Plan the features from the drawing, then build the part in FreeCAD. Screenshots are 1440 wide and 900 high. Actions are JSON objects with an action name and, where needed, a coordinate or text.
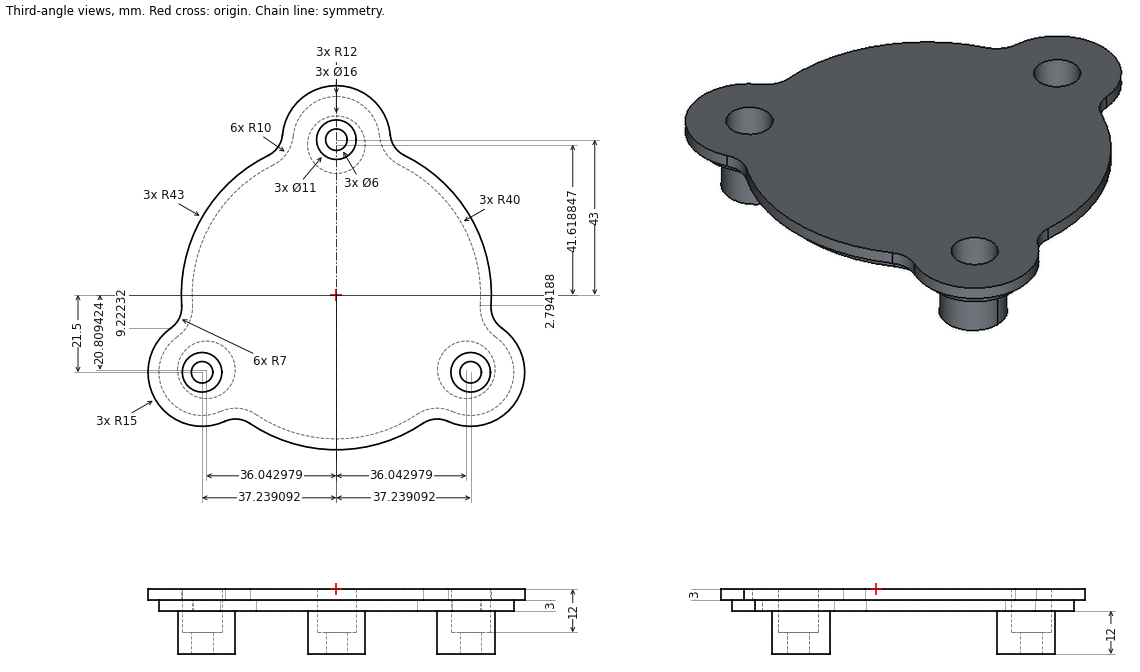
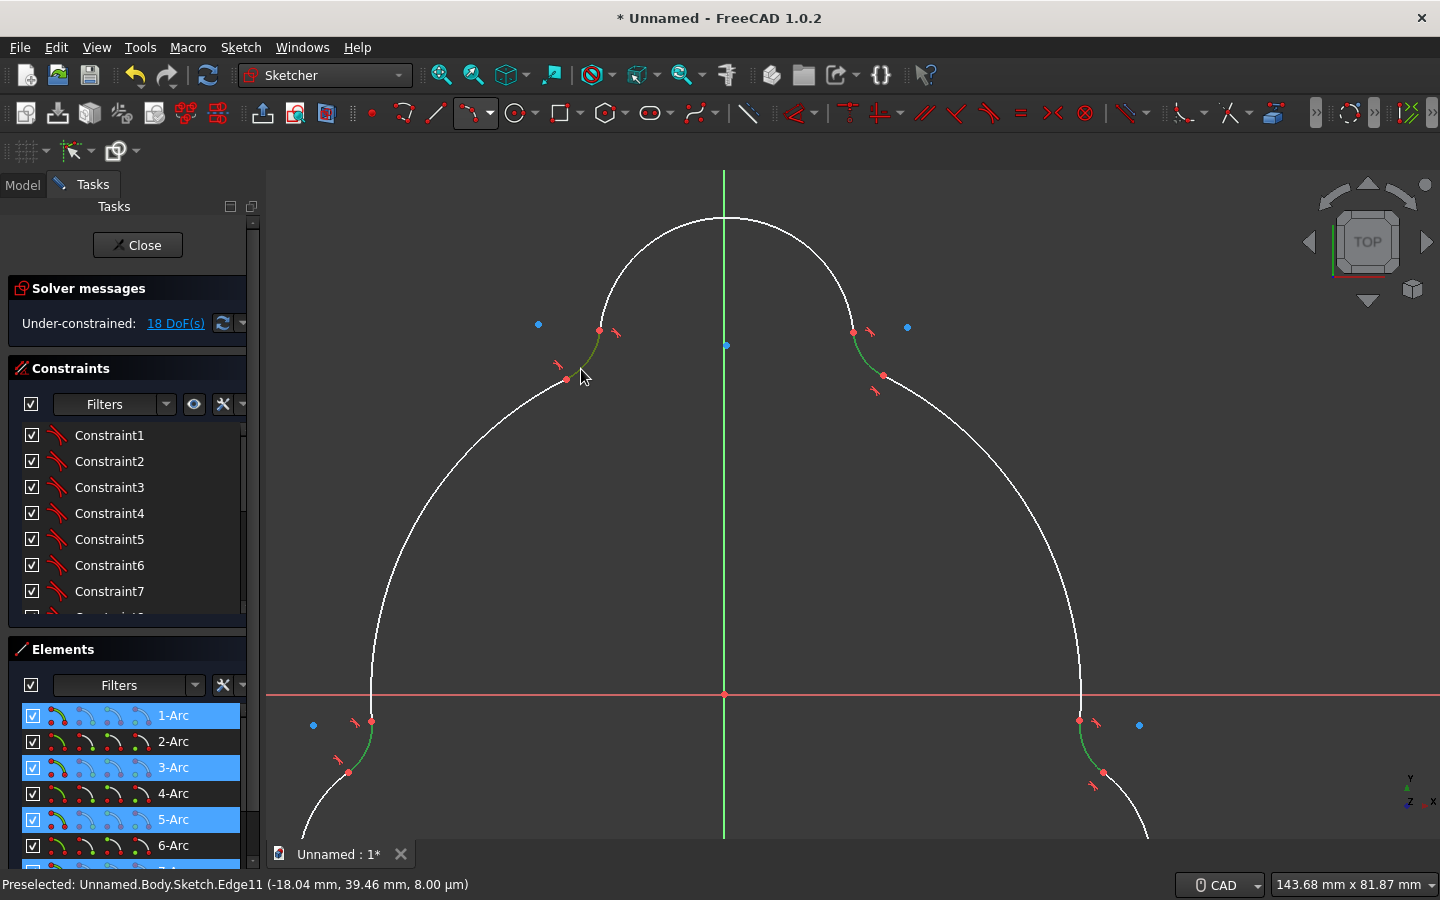
{"action": "left_click", "coordinate": [1022, 114]}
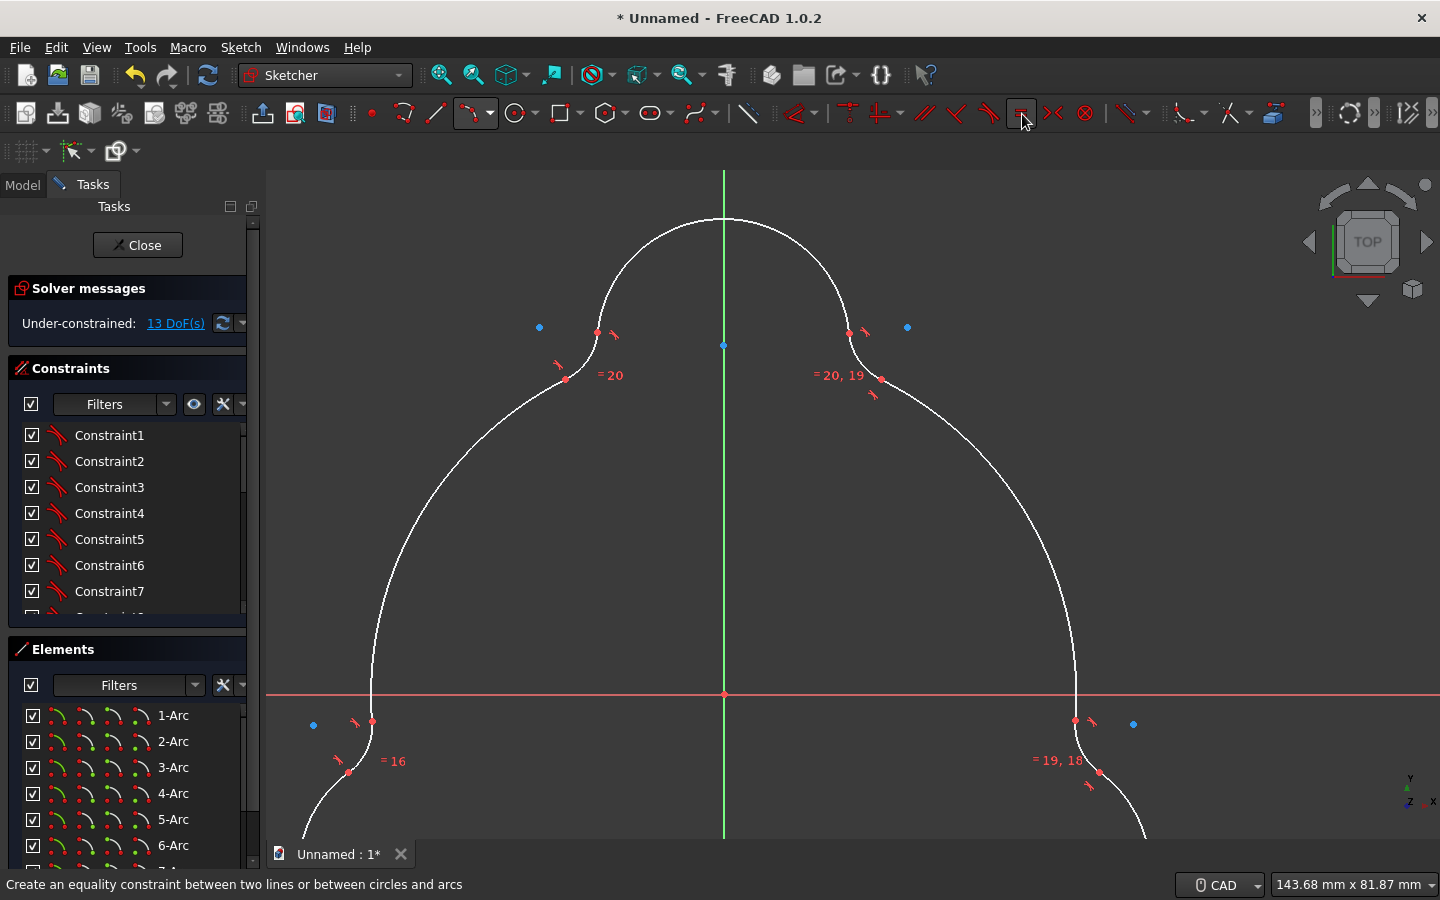
{"action": "scroll", "coordinate": [858, 347], "scroll_direction": "down", "scroll_amount": 3}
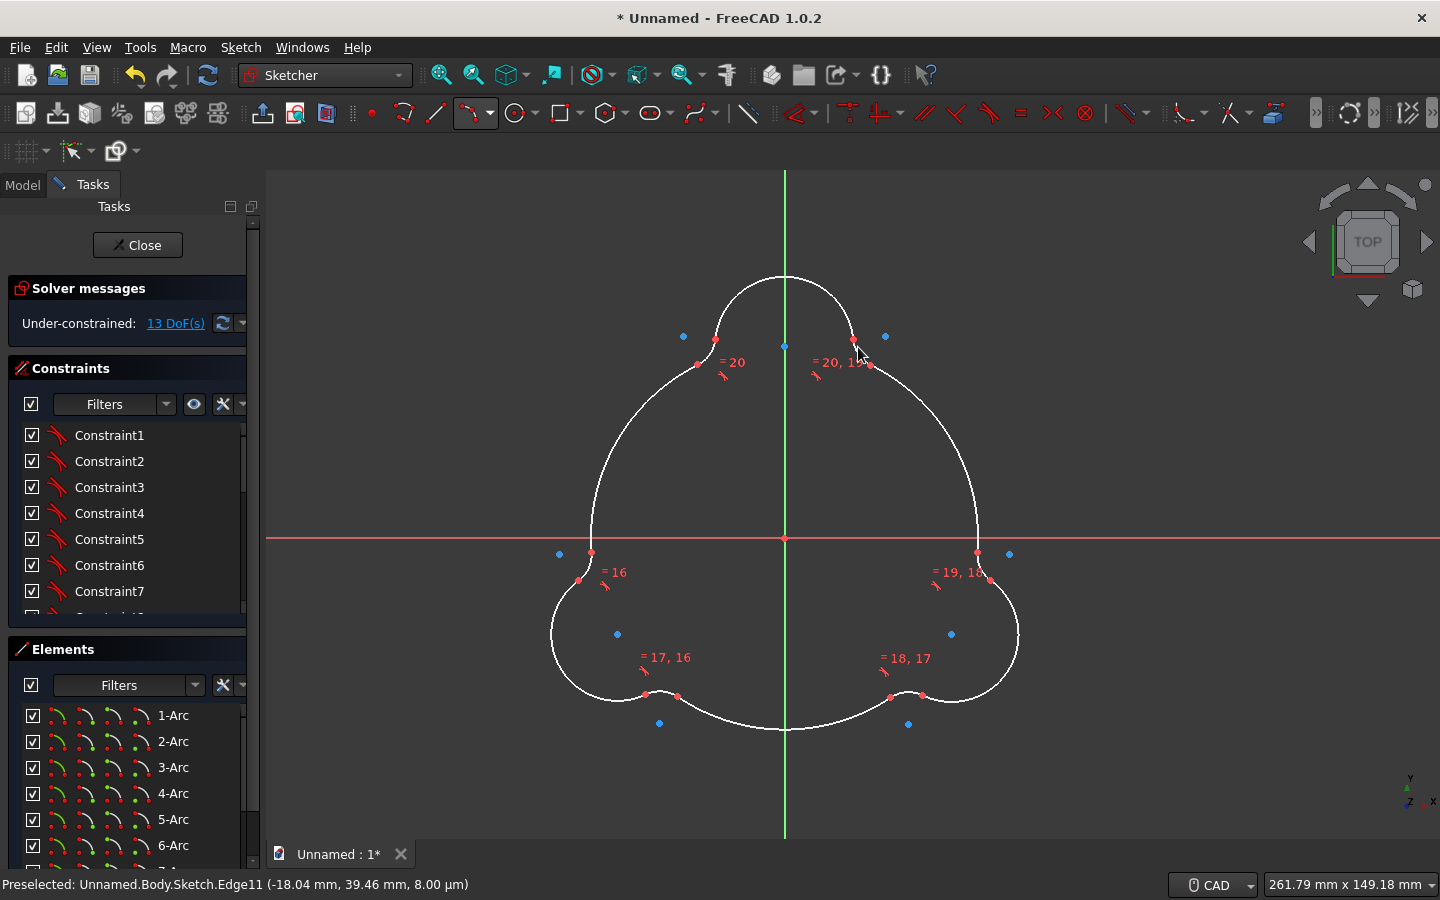
{"action": "left_click", "coordinate": [551, 631]}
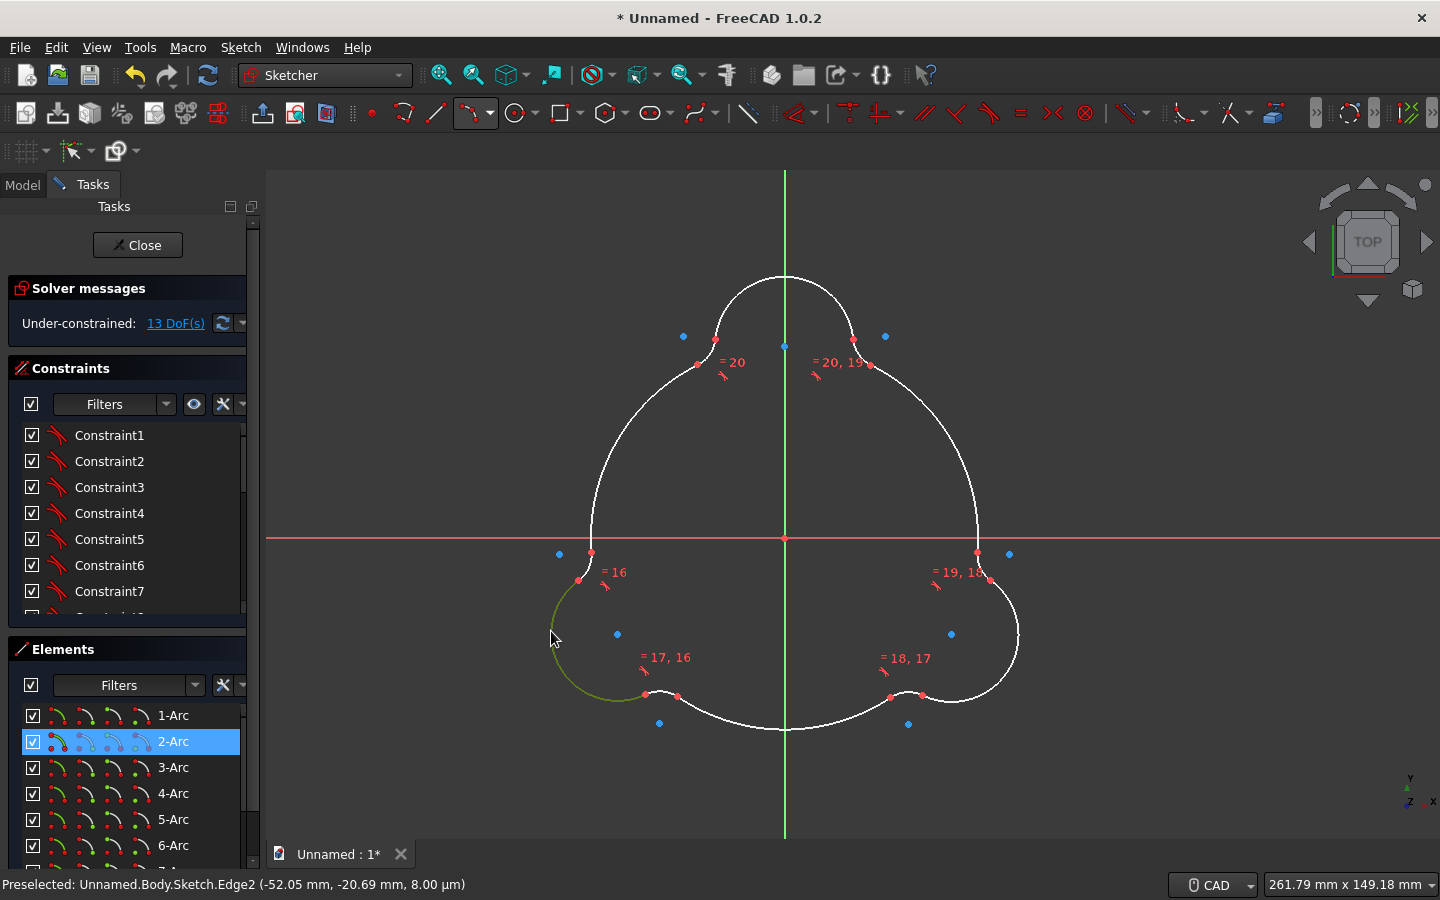
{"action": "left_click", "coordinate": [980, 695]}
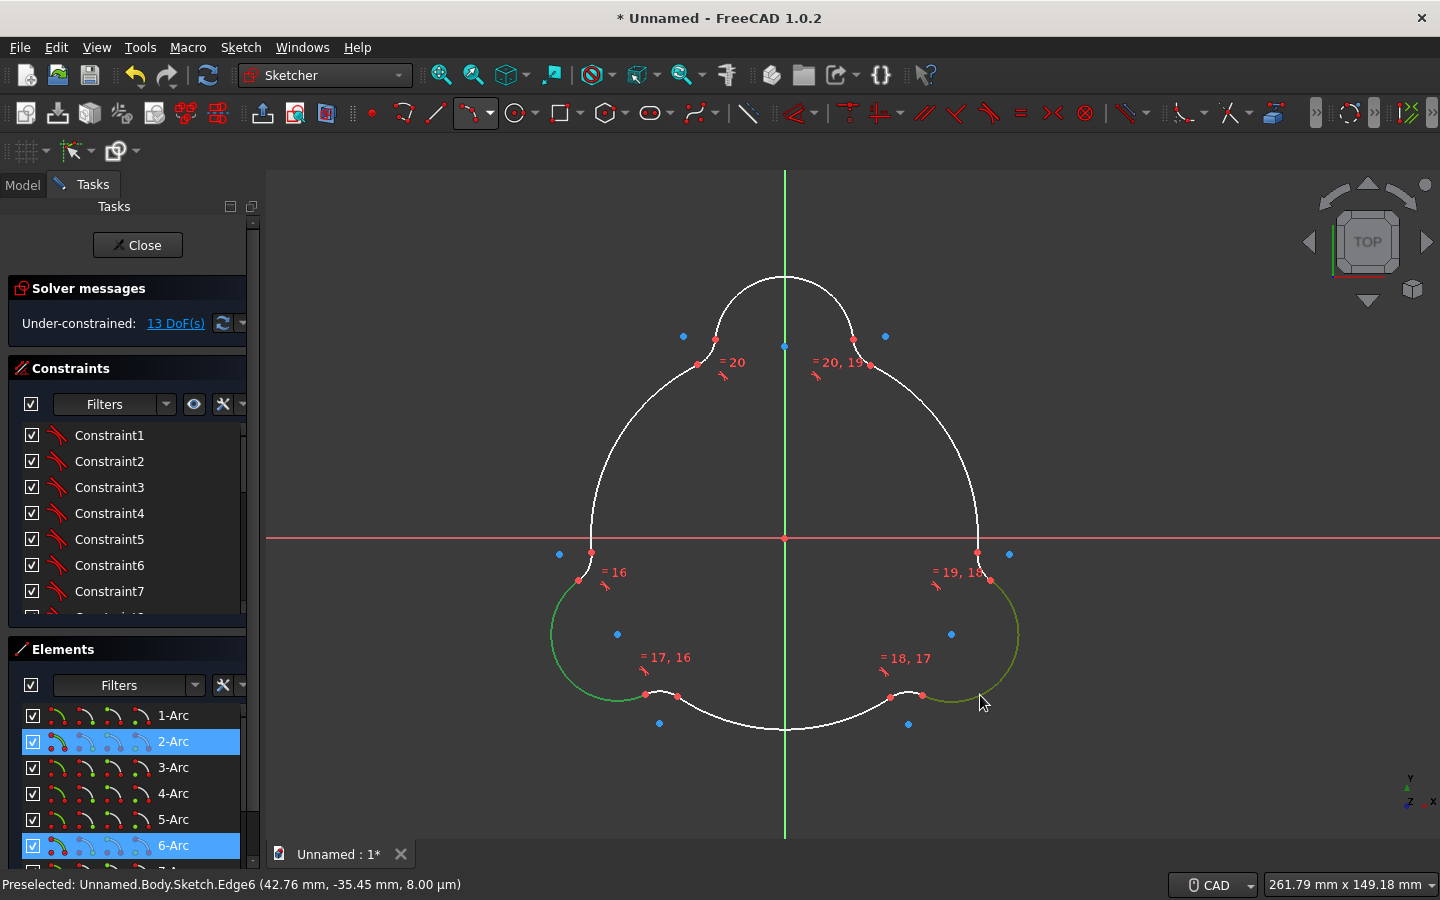
{"action": "left_click", "coordinate": [823, 289]}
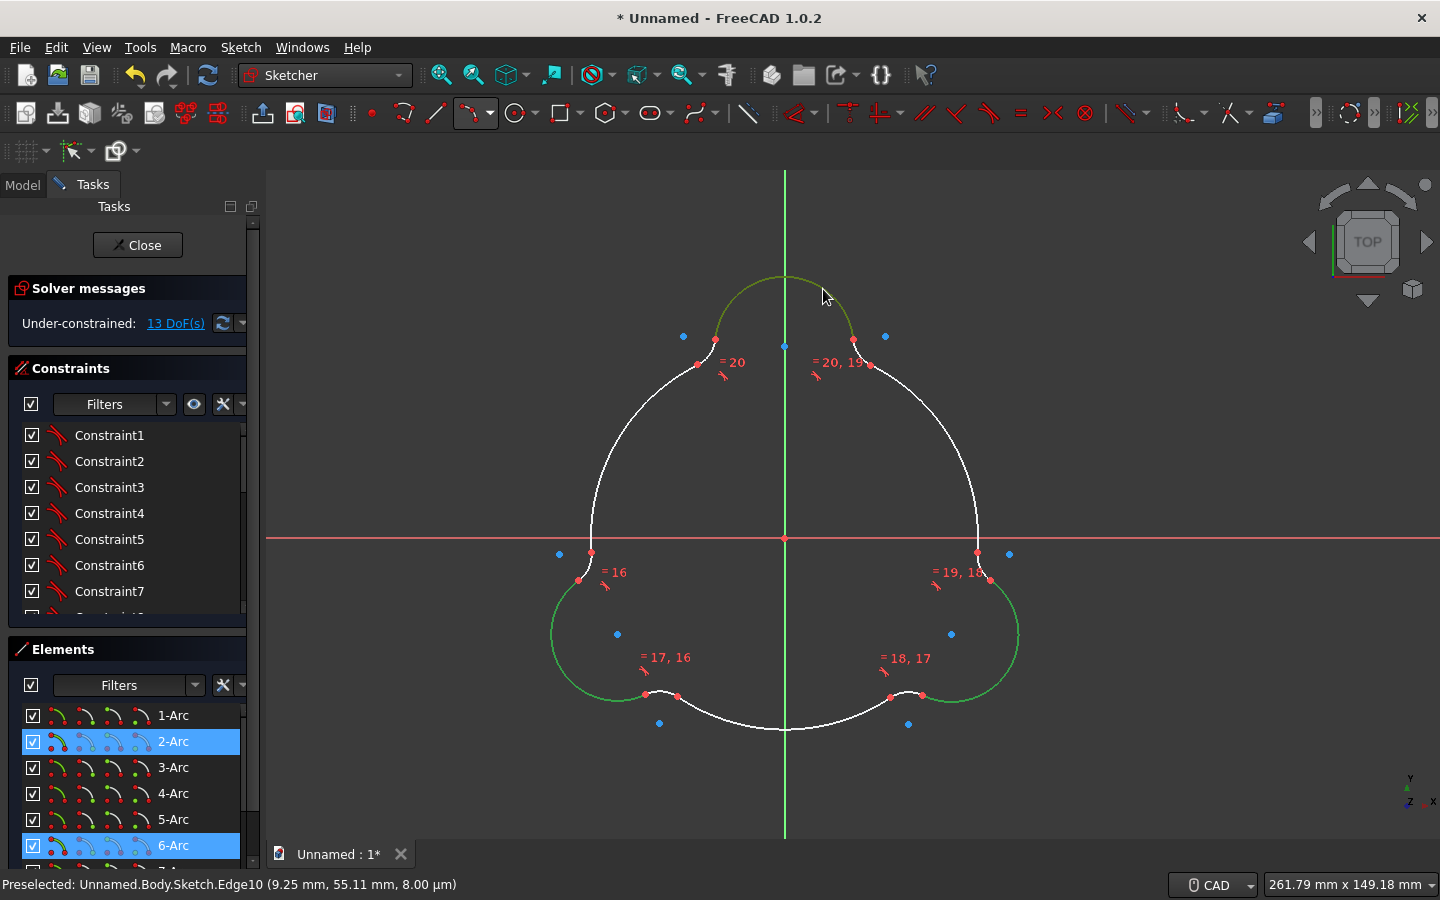
{"action": "left_click", "coordinate": [1022, 114]}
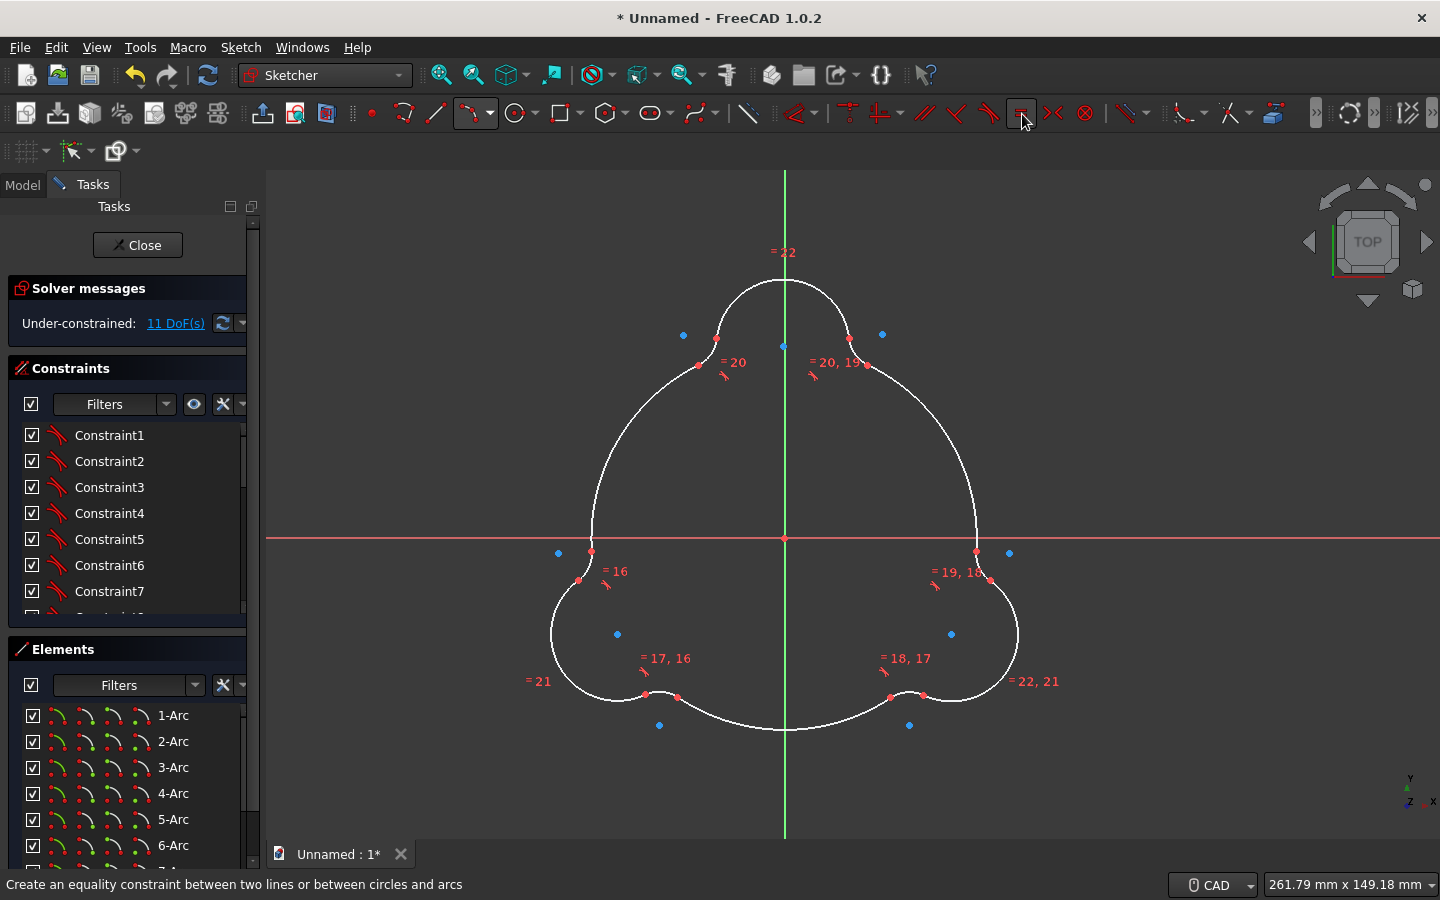
{"action": "left_click", "coordinate": [740, 725]}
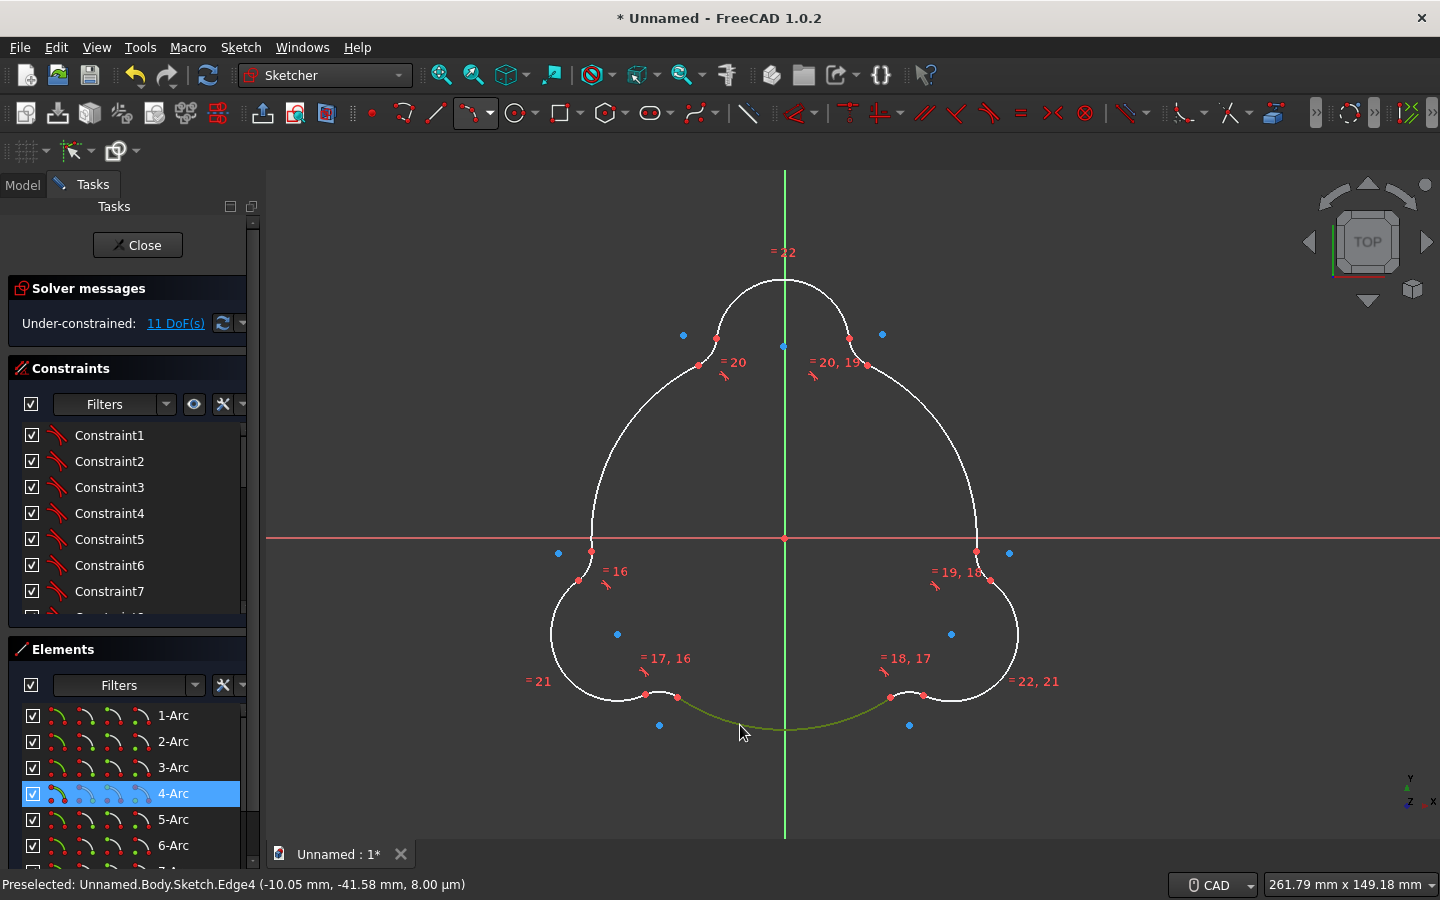
{"action": "left_click", "coordinate": [969, 483]}